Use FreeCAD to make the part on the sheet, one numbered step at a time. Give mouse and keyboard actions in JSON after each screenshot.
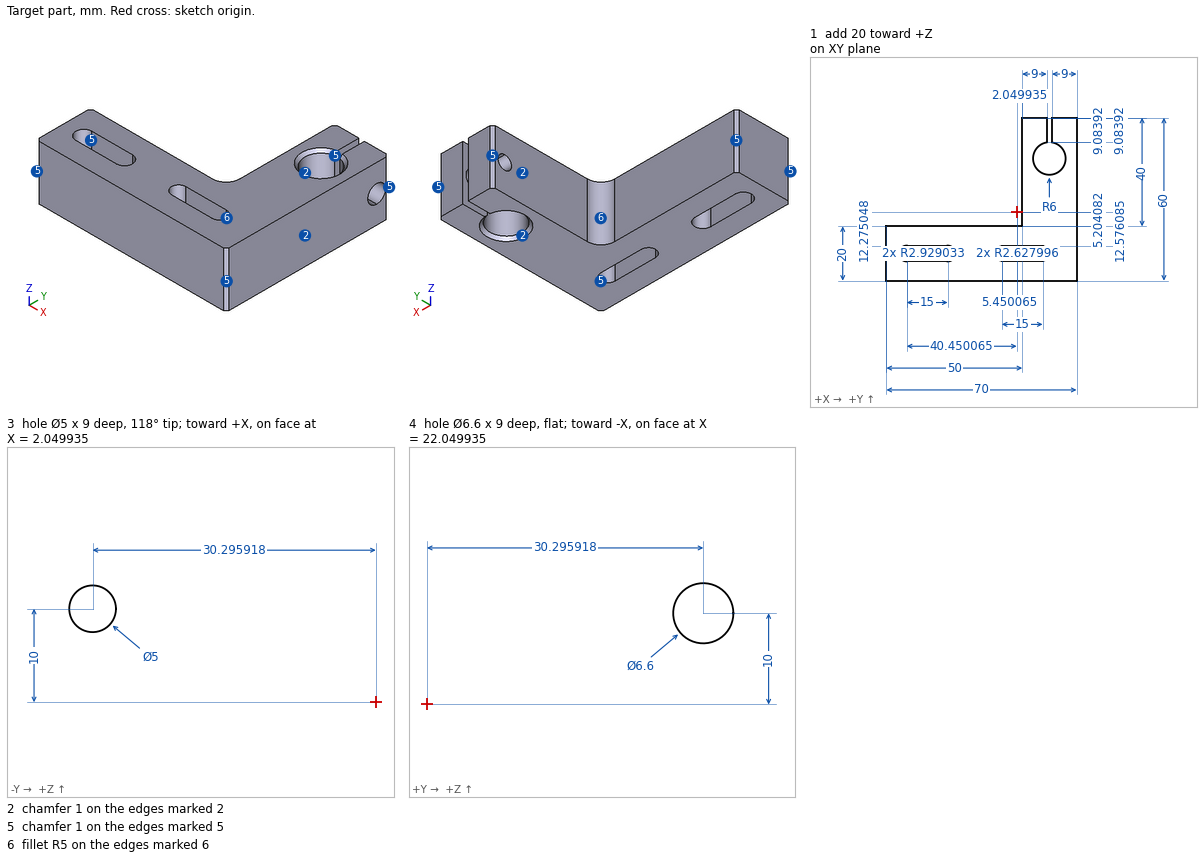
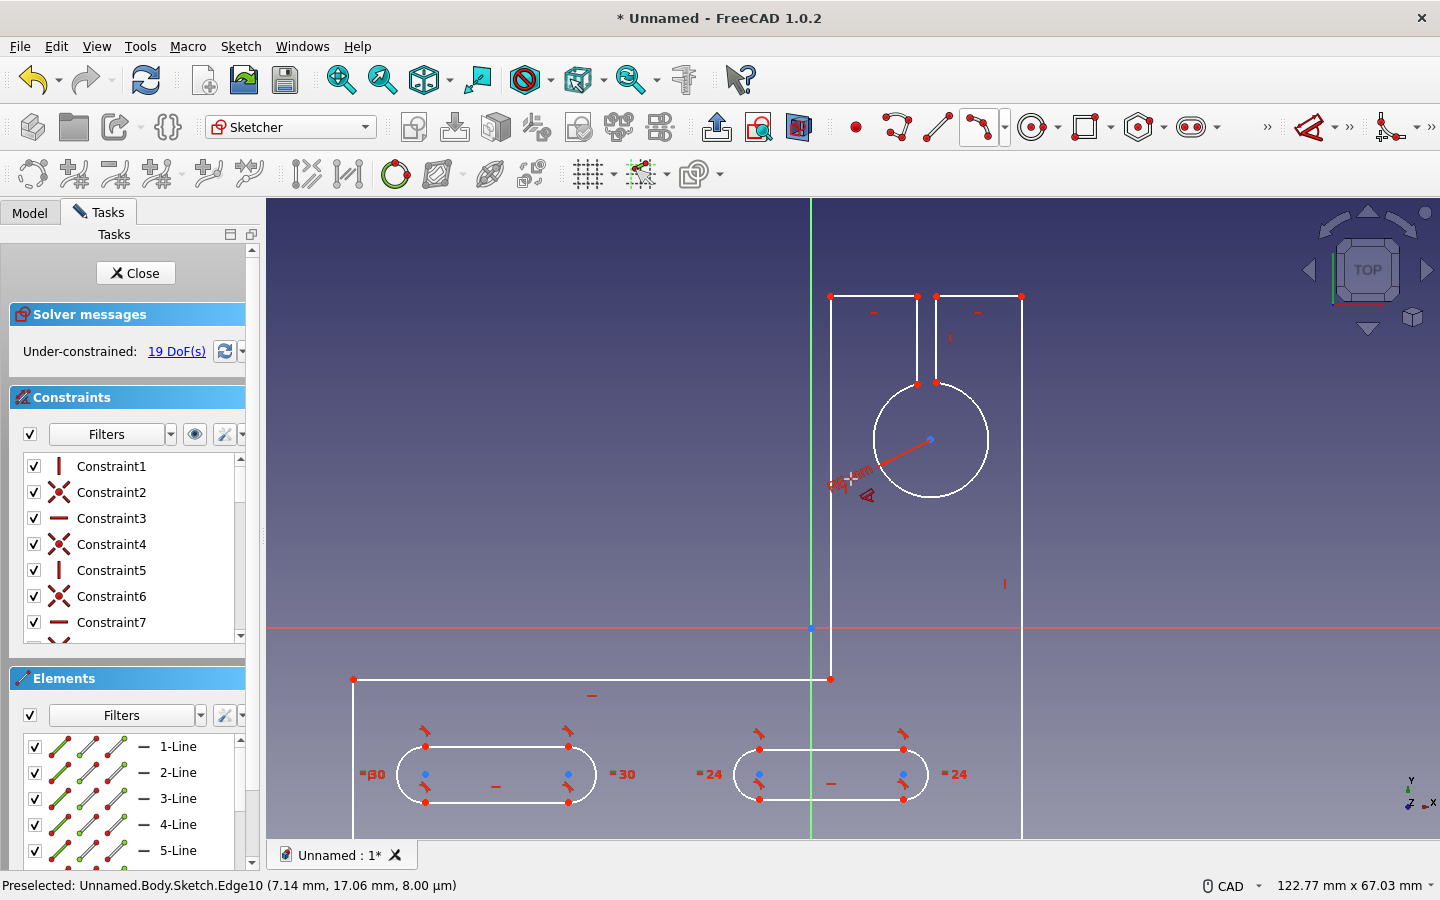
{"action": "scroll", "coordinate": [739, 760], "scroll_direction": "up", "scroll_amount": 3}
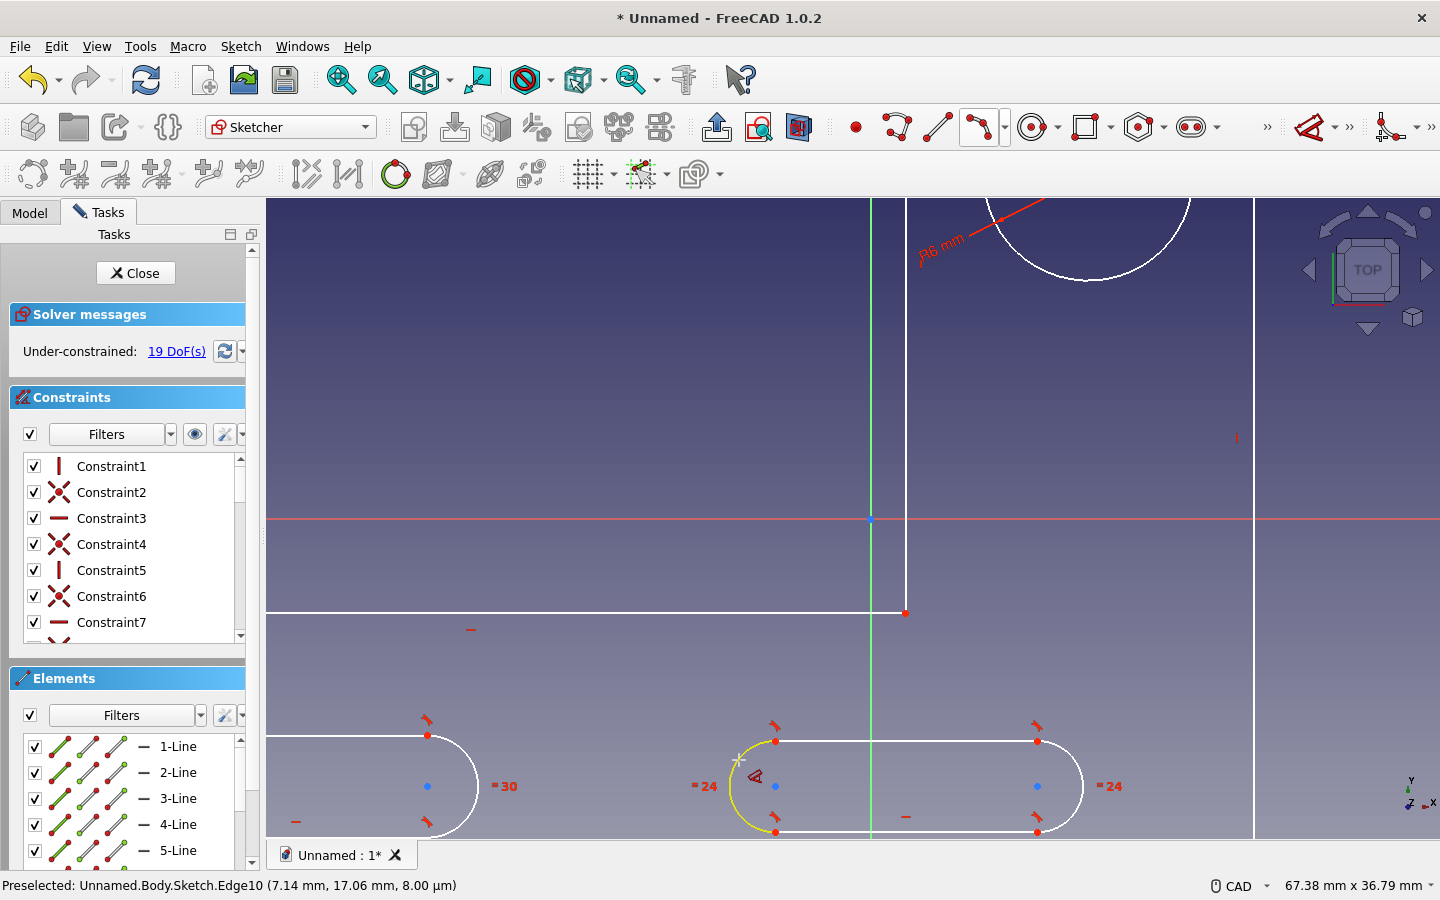
{"action": "left_click", "coordinate": [738, 760]}
{"action": "left_click", "coordinate": [712, 741]}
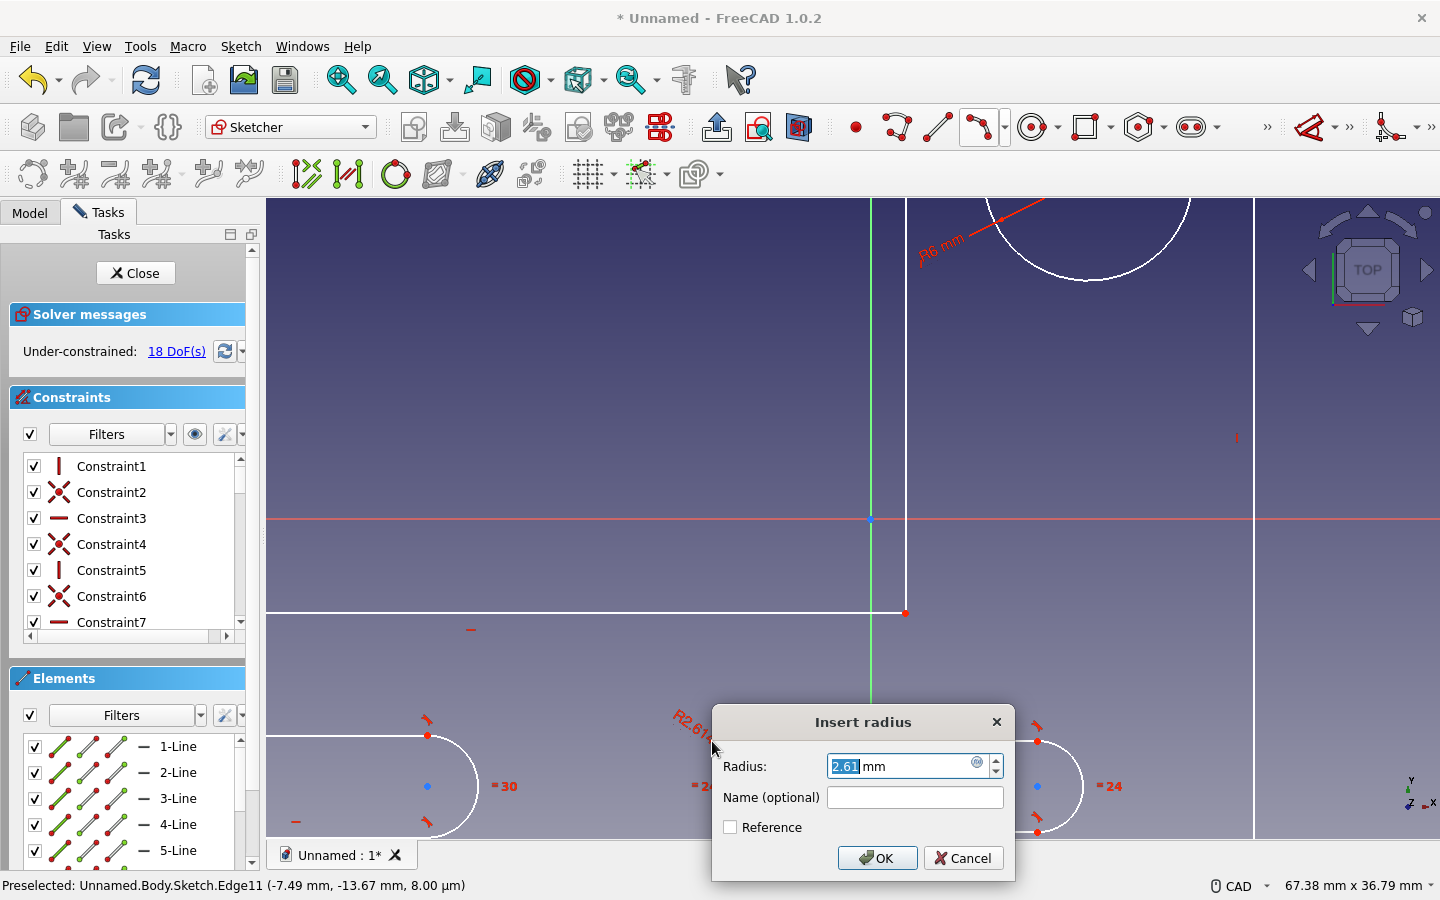
{"action": "type", "text": "2.627996"}
{"action": "key", "text": "Return"}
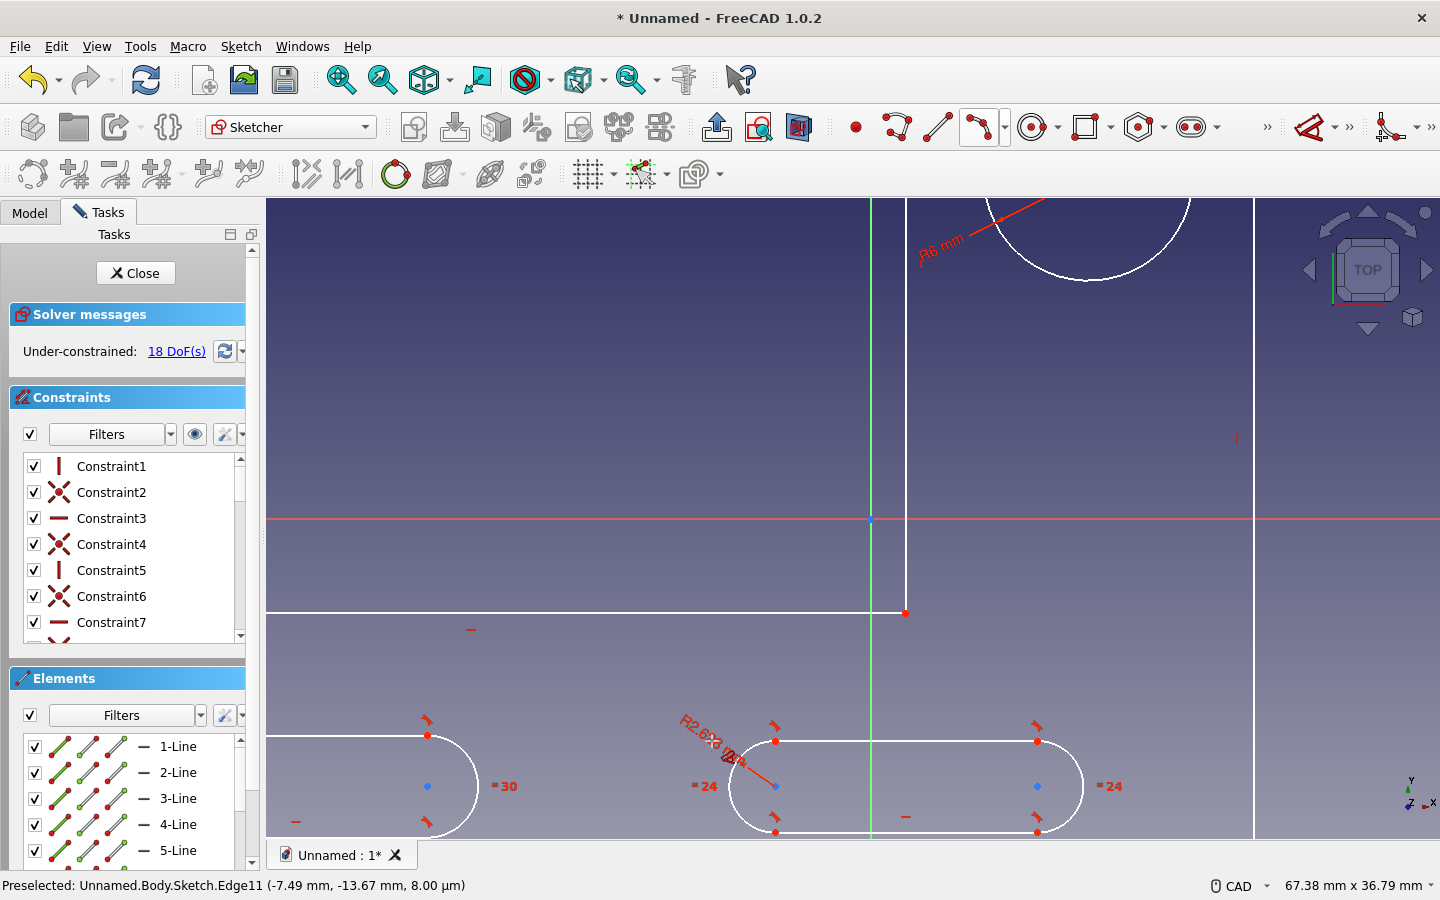
{"action": "scroll", "coordinate": [866, 567], "scroll_direction": "down", "scroll_amount": 5}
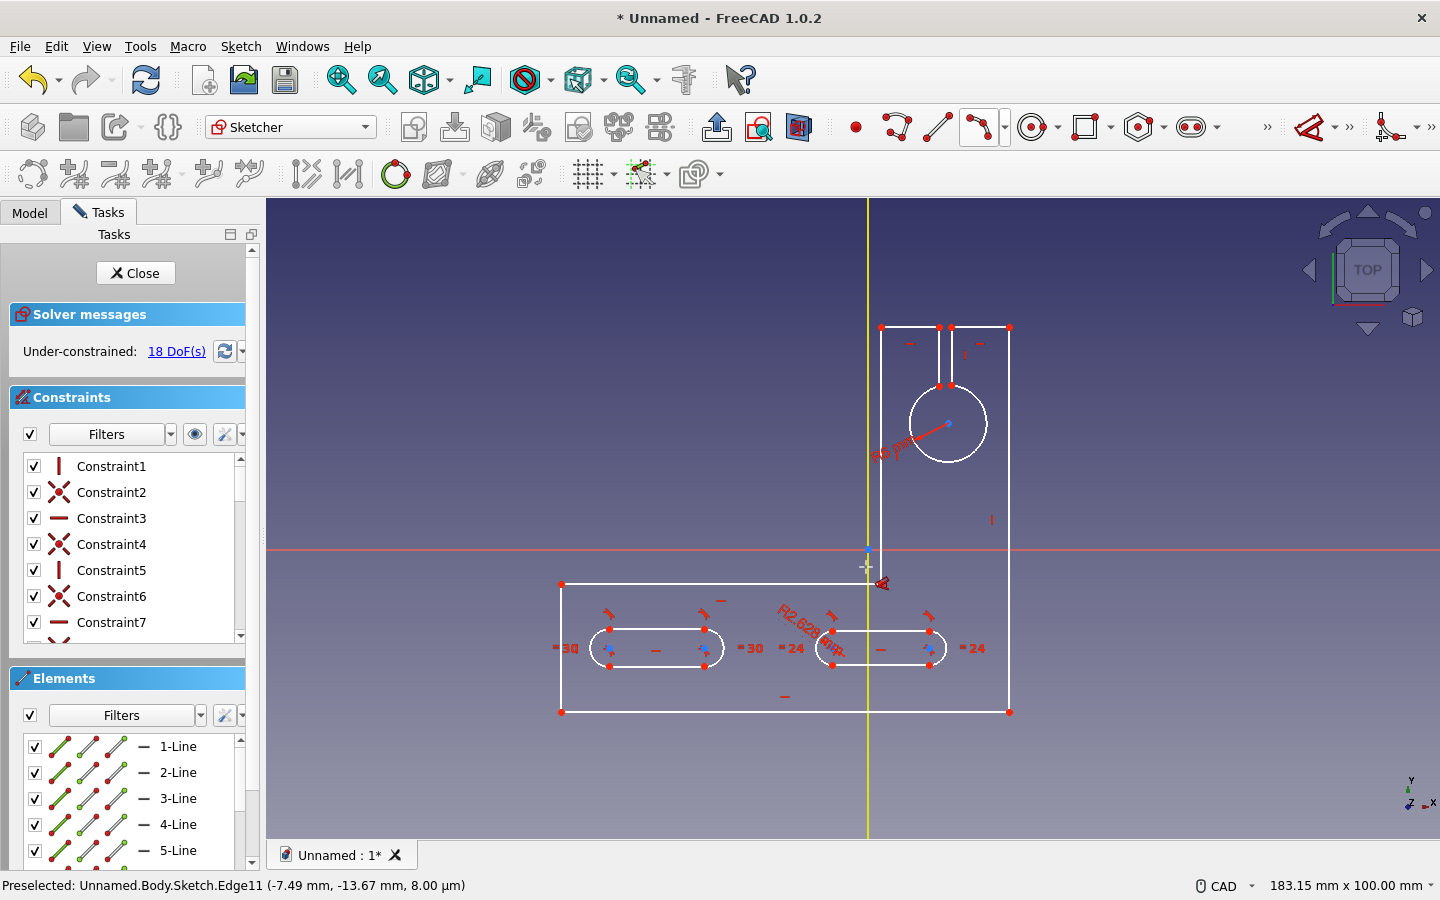
{"action": "scroll", "coordinate": [594, 637], "scroll_direction": "up", "scroll_amount": 4}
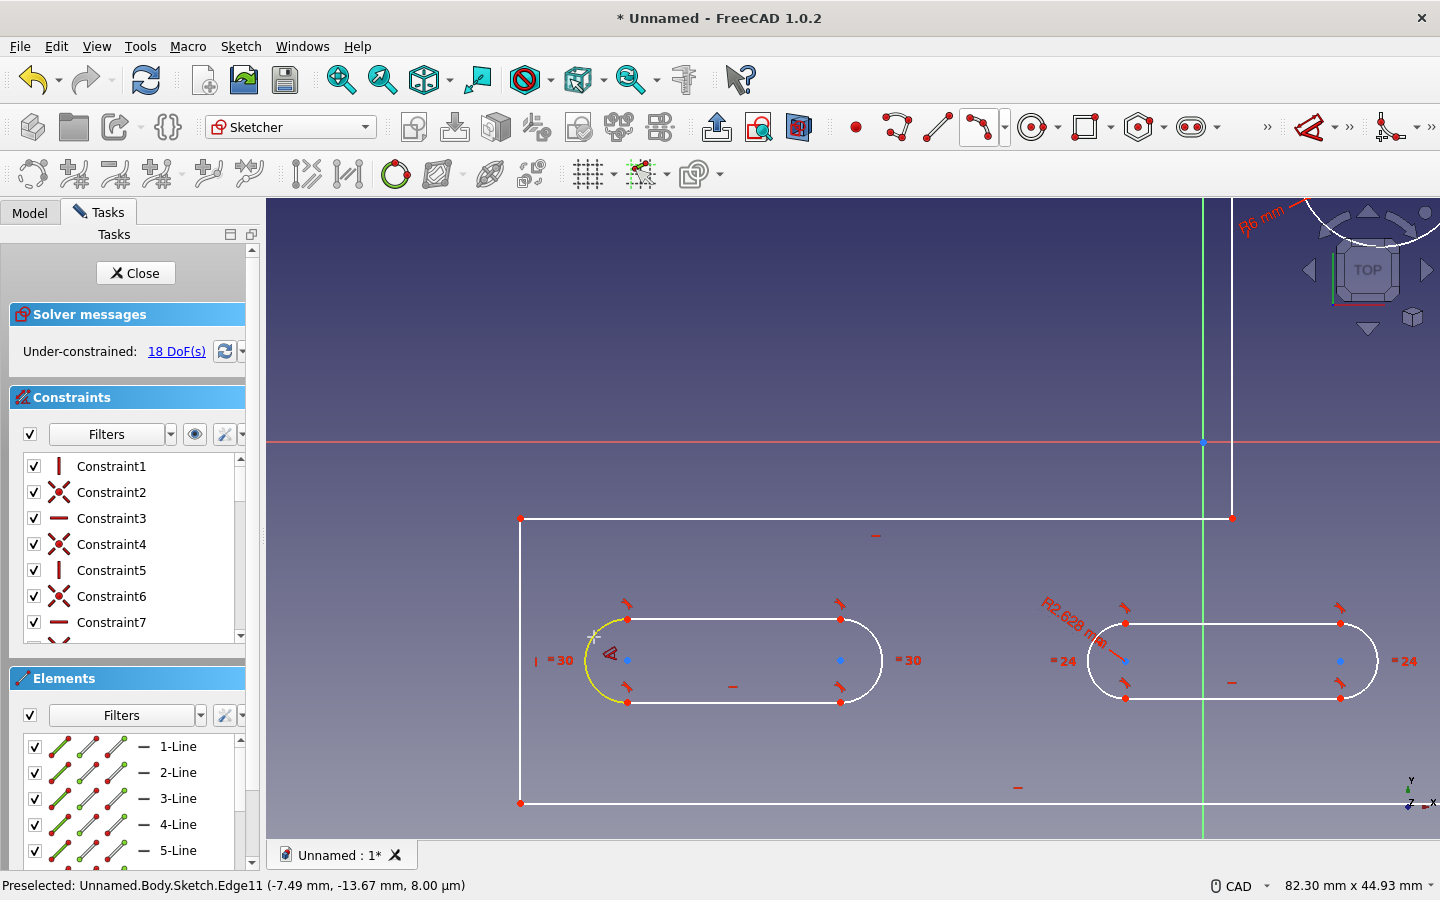
{"action": "left_click", "coordinate": [593, 636]}
{"action": "left_click", "coordinate": [567, 617]}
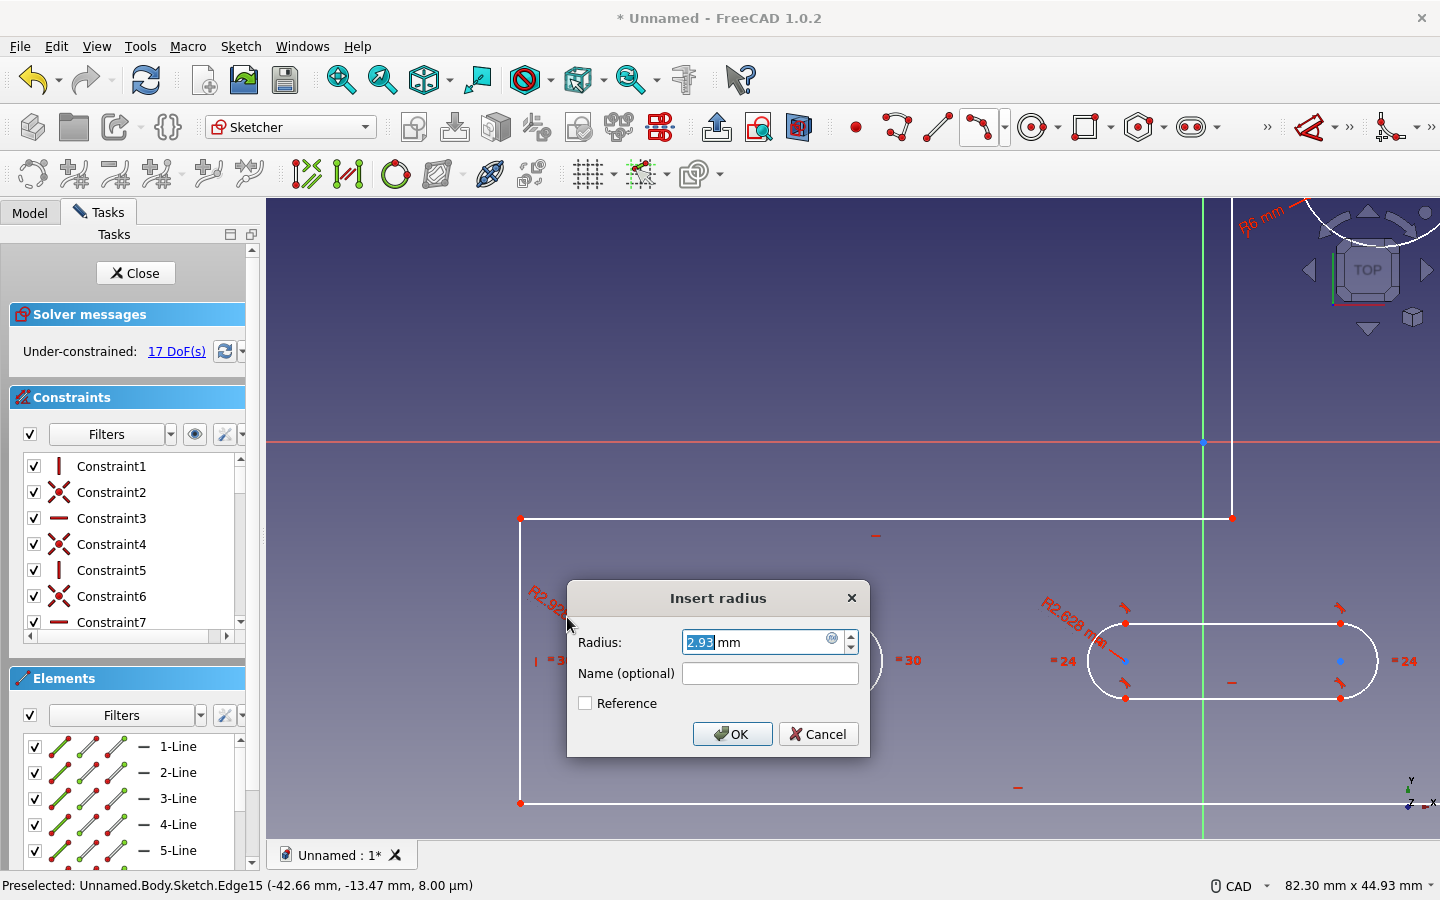
{"action": "type", "text": "2.929033"}
{"action": "key", "text": "Return"}